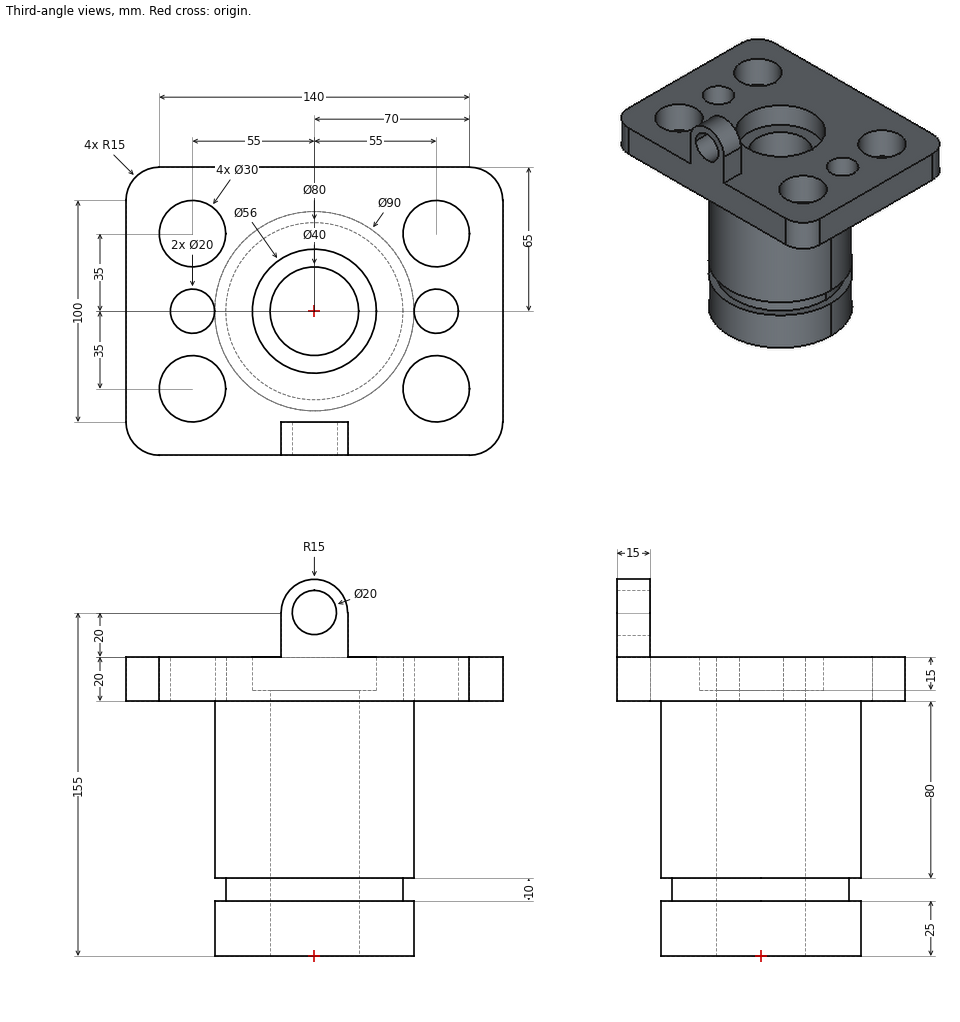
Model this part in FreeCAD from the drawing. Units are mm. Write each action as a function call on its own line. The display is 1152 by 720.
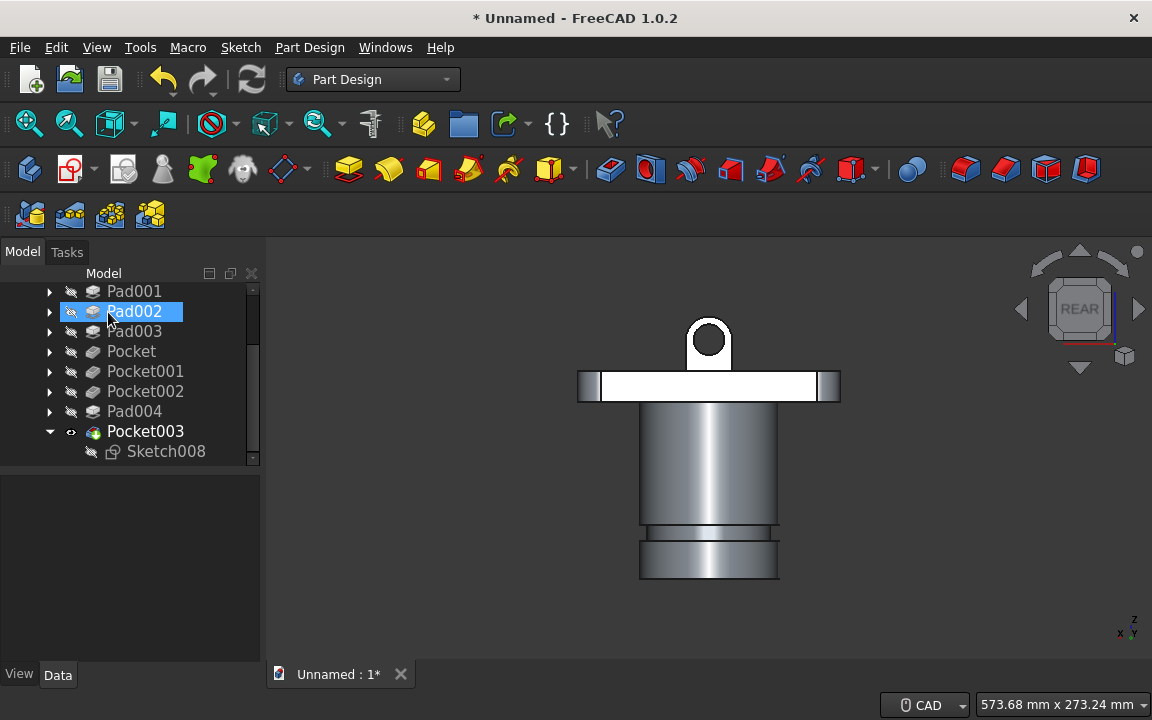
key(0)